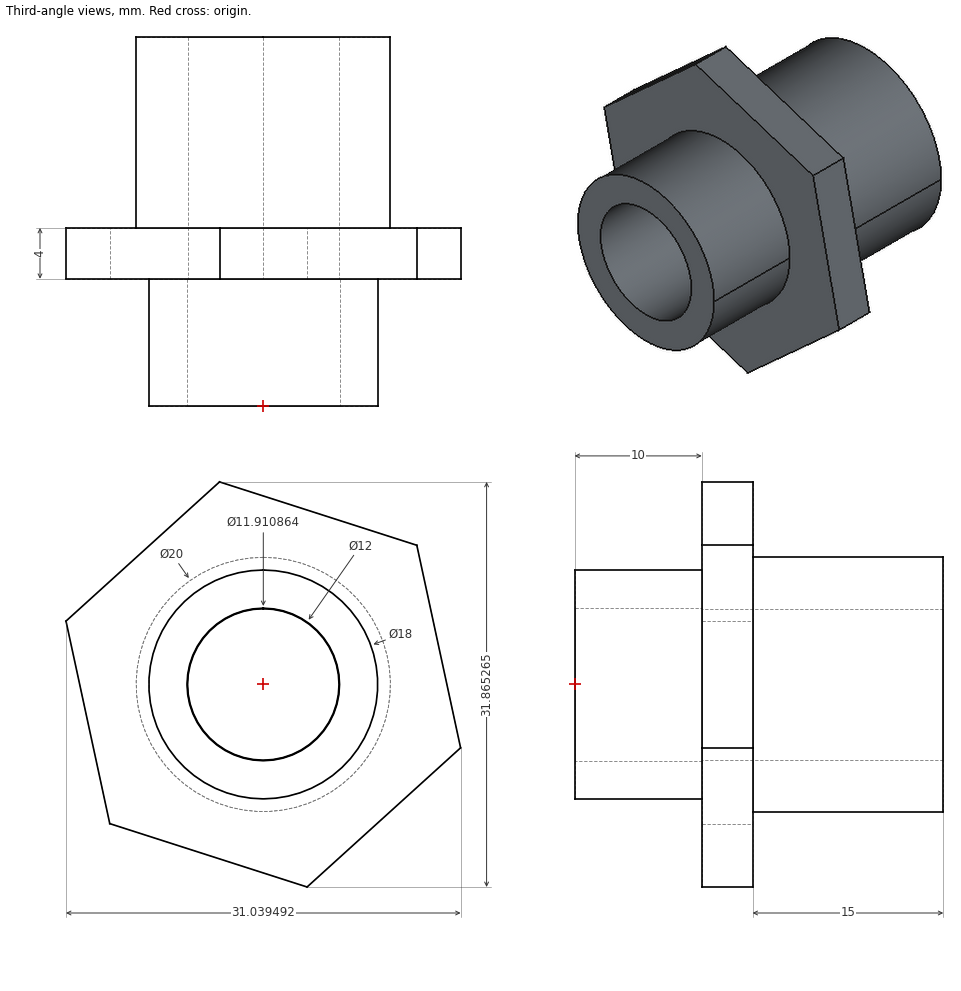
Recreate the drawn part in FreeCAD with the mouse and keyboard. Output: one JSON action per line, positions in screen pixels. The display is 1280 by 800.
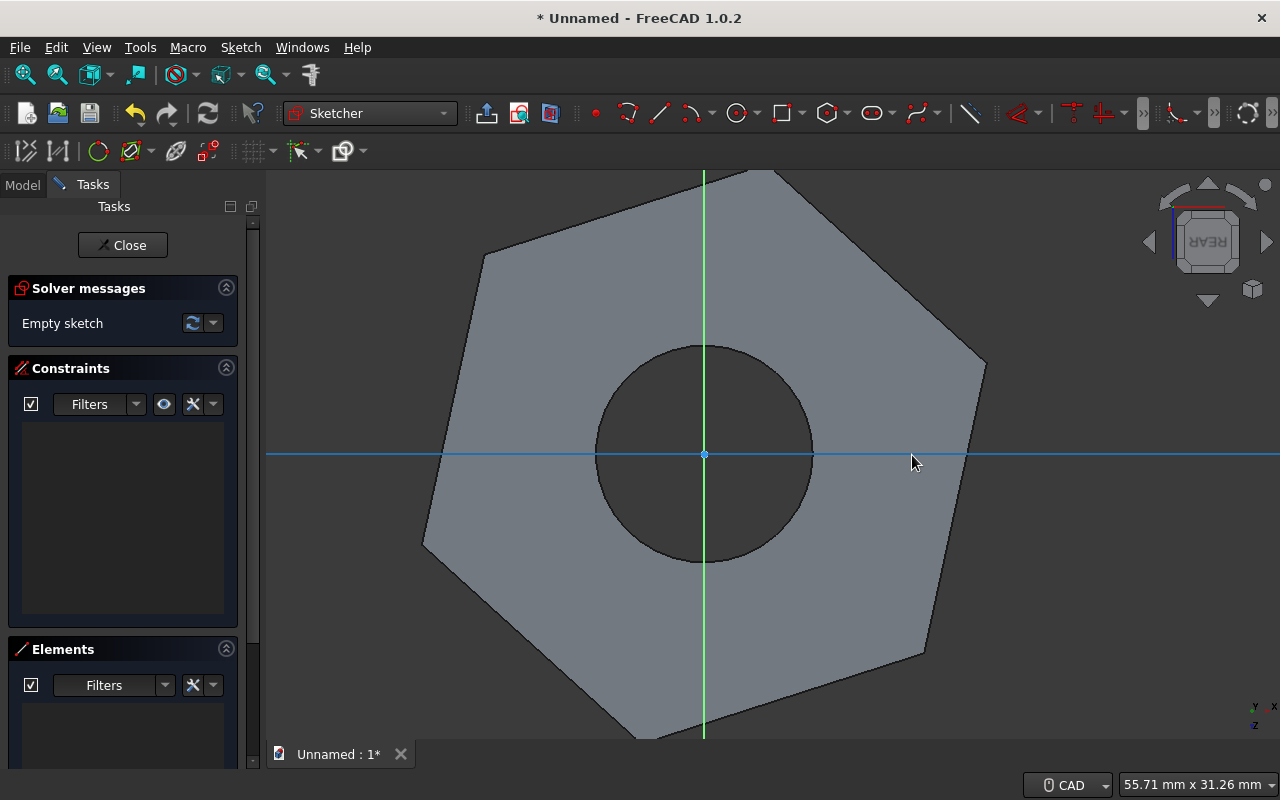
{"action": "left_click", "coordinate": [738, 114]}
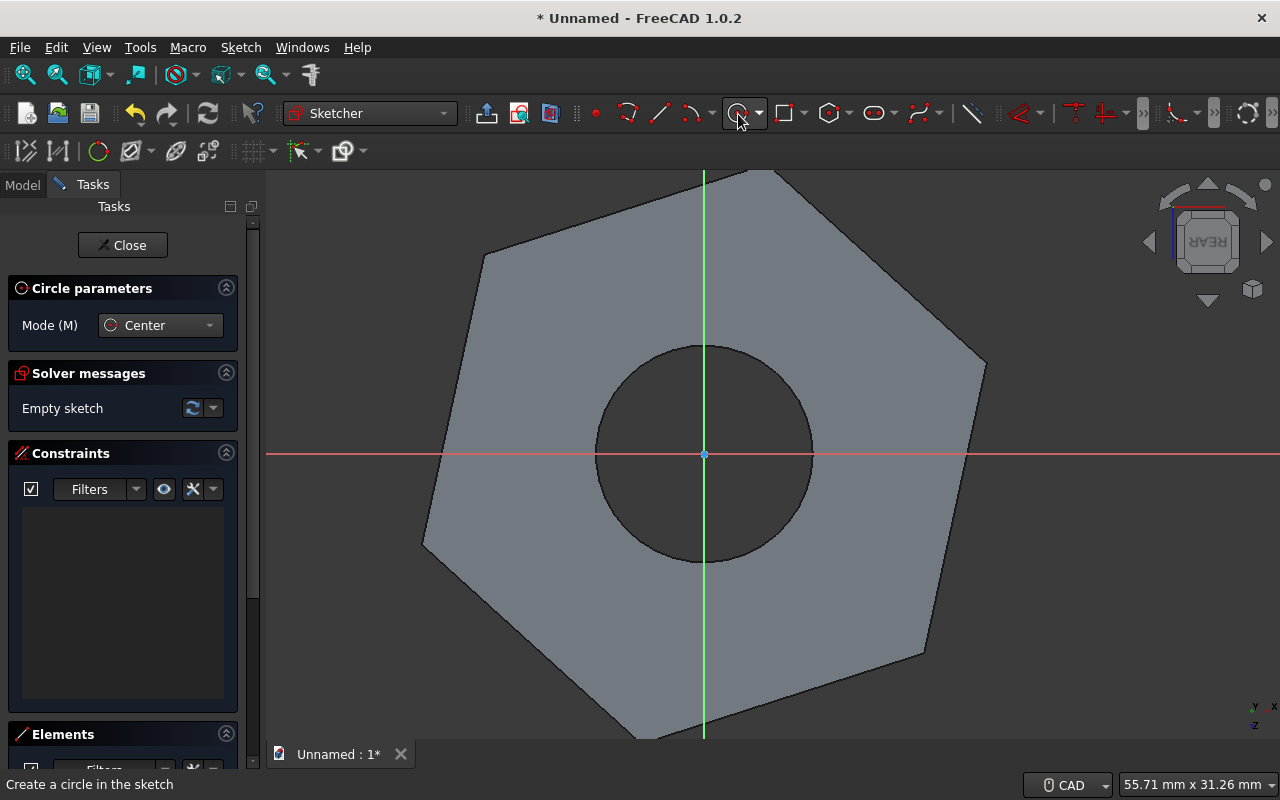
{"action": "left_click", "coordinate": [704, 454]}
{"action": "mouse_move", "coordinate": [833, 325]}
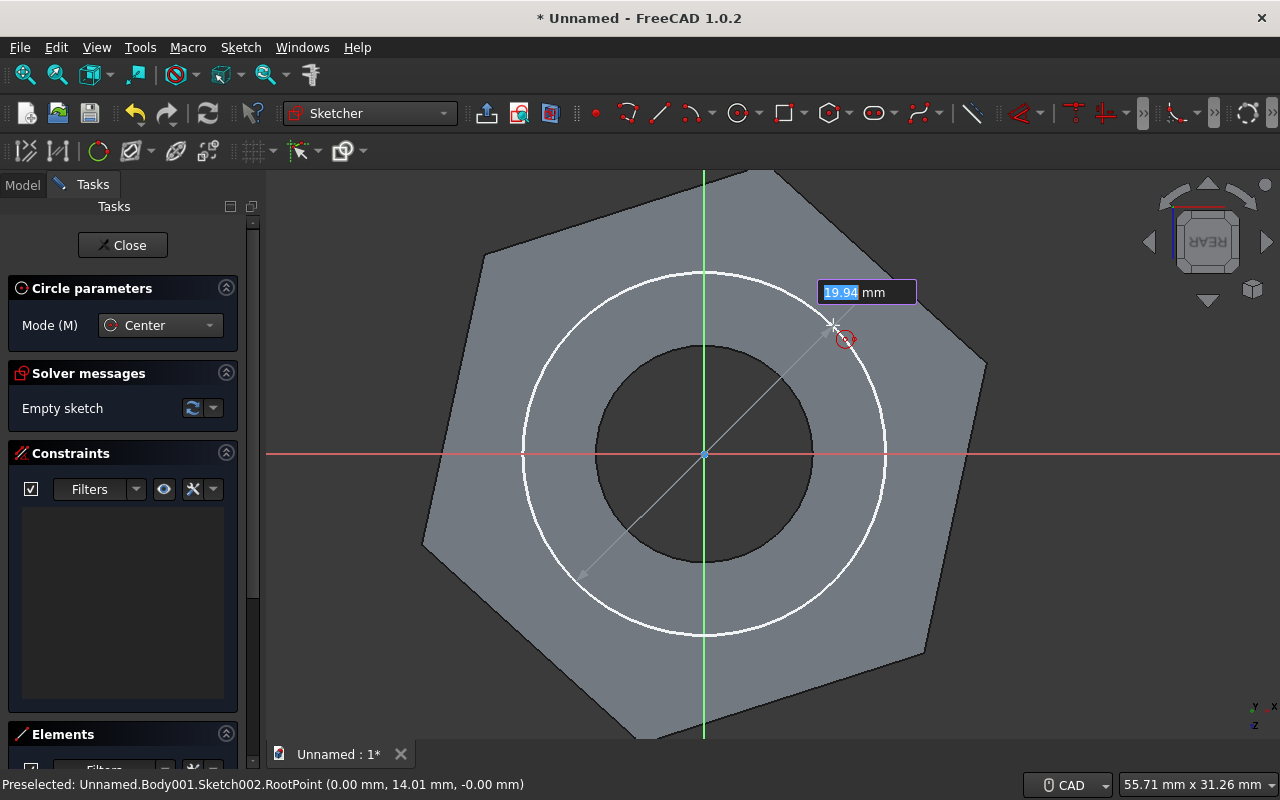
{"action": "type", "text": "20"}
{"action": "key", "text": "Return"}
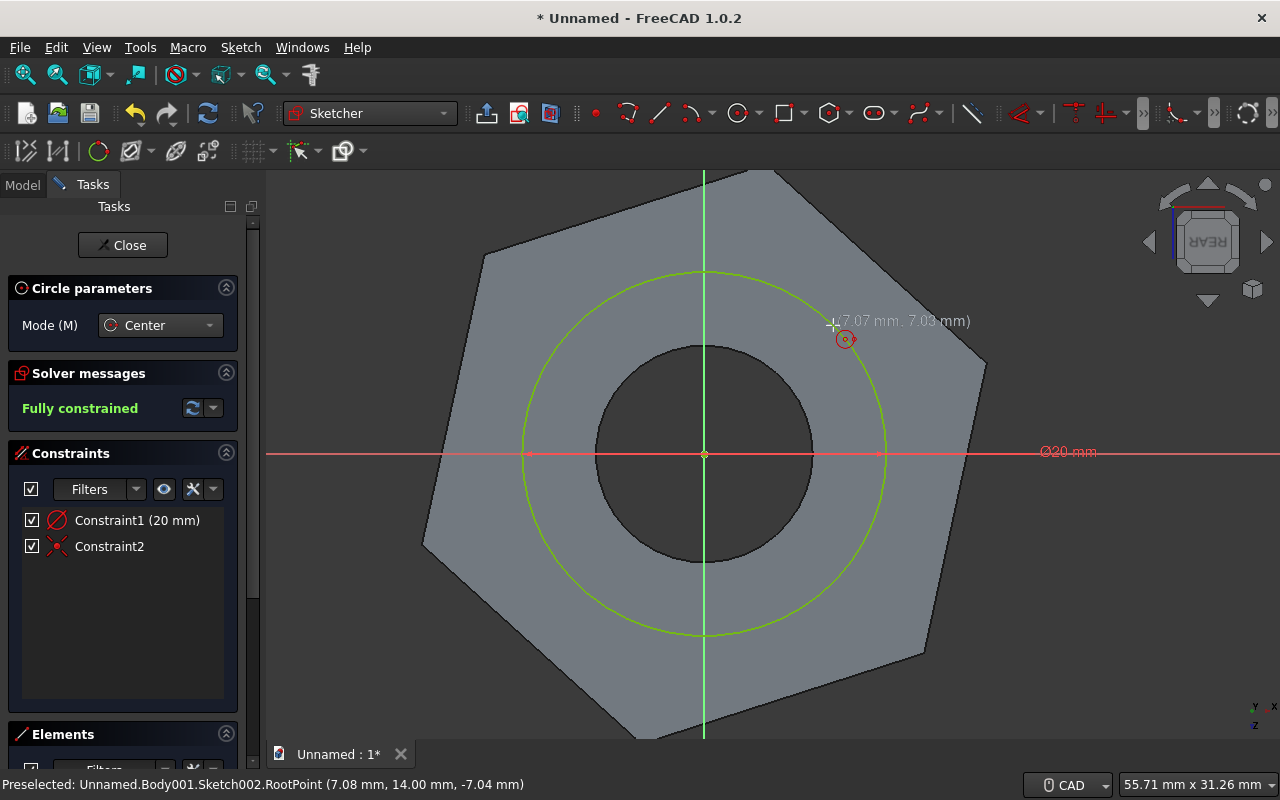
{"action": "left_click", "coordinate": [704, 454]}
{"action": "mouse_move", "coordinate": [781, 377]}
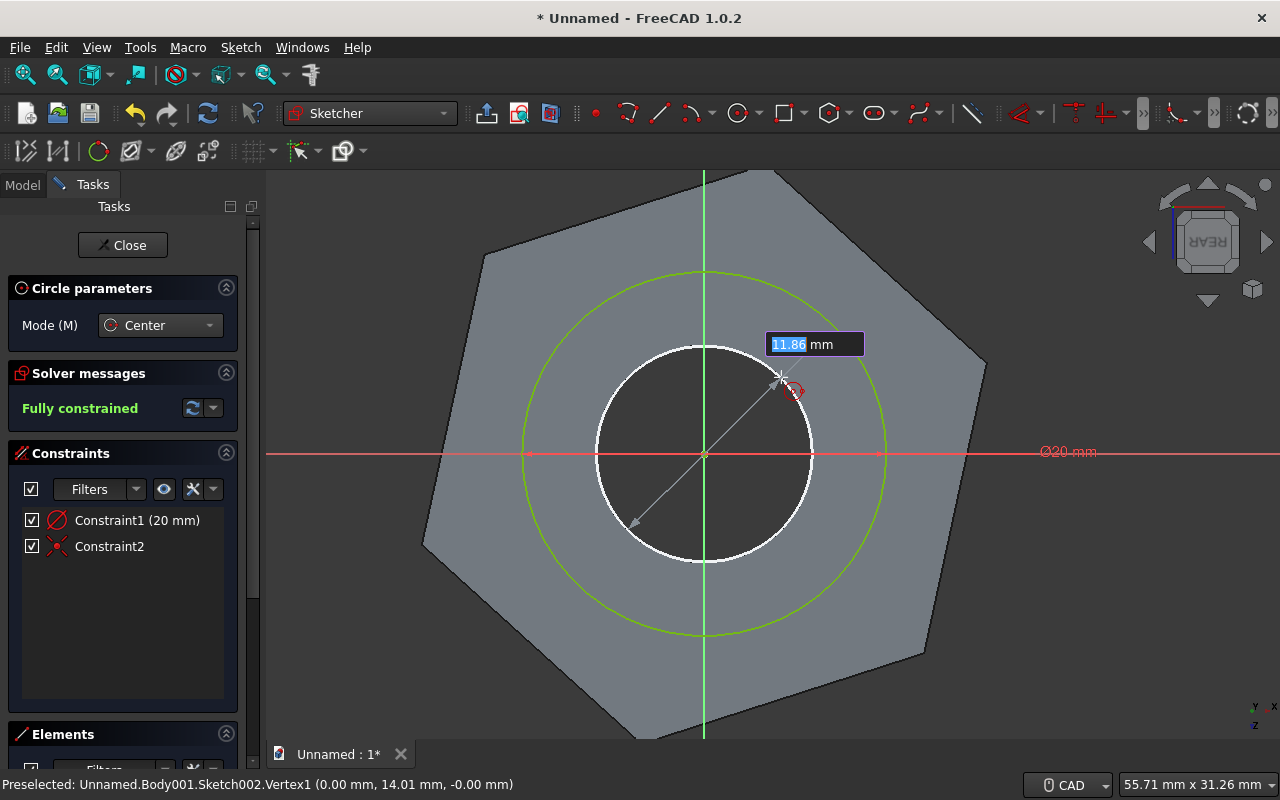
{"action": "type", "text": "11.910864"}
{"action": "key", "text": "Return"}
{"action": "key", "text": "Escape"}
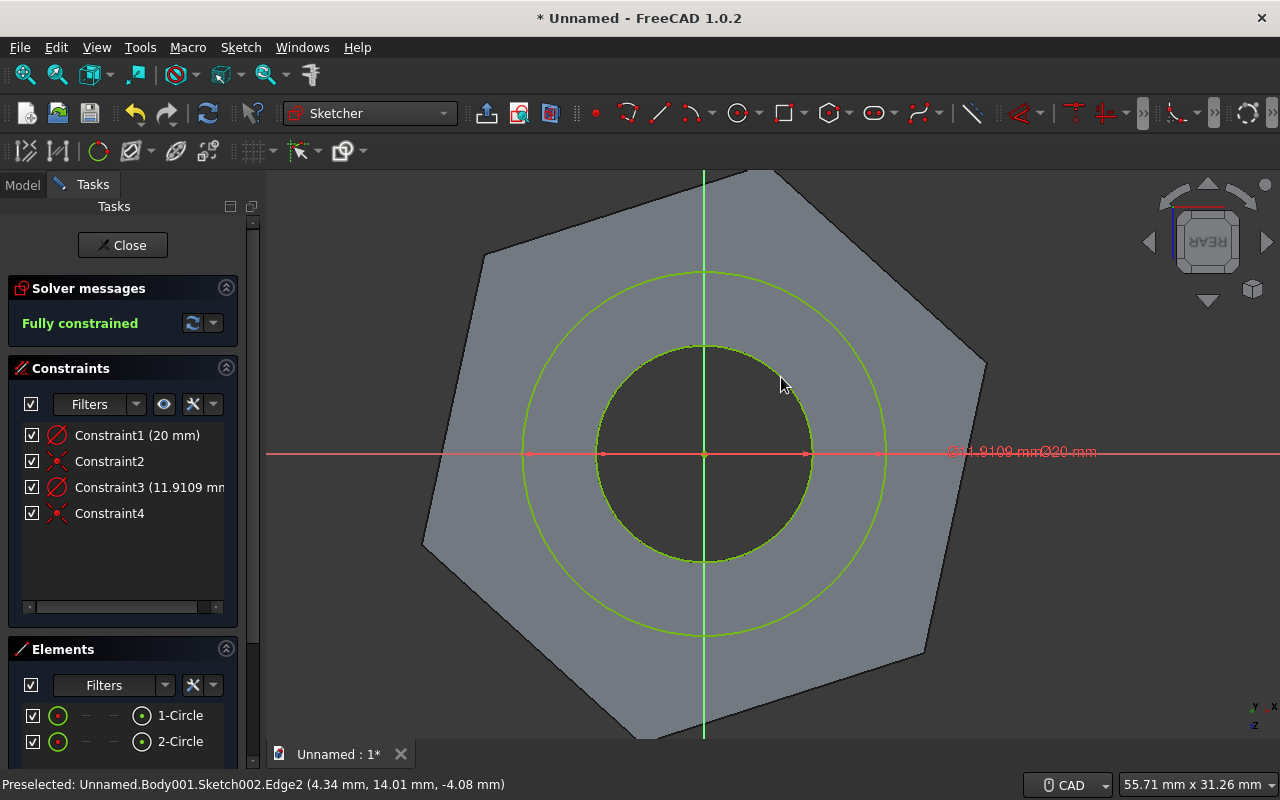
{"action": "left_click", "coordinate": [123, 245]}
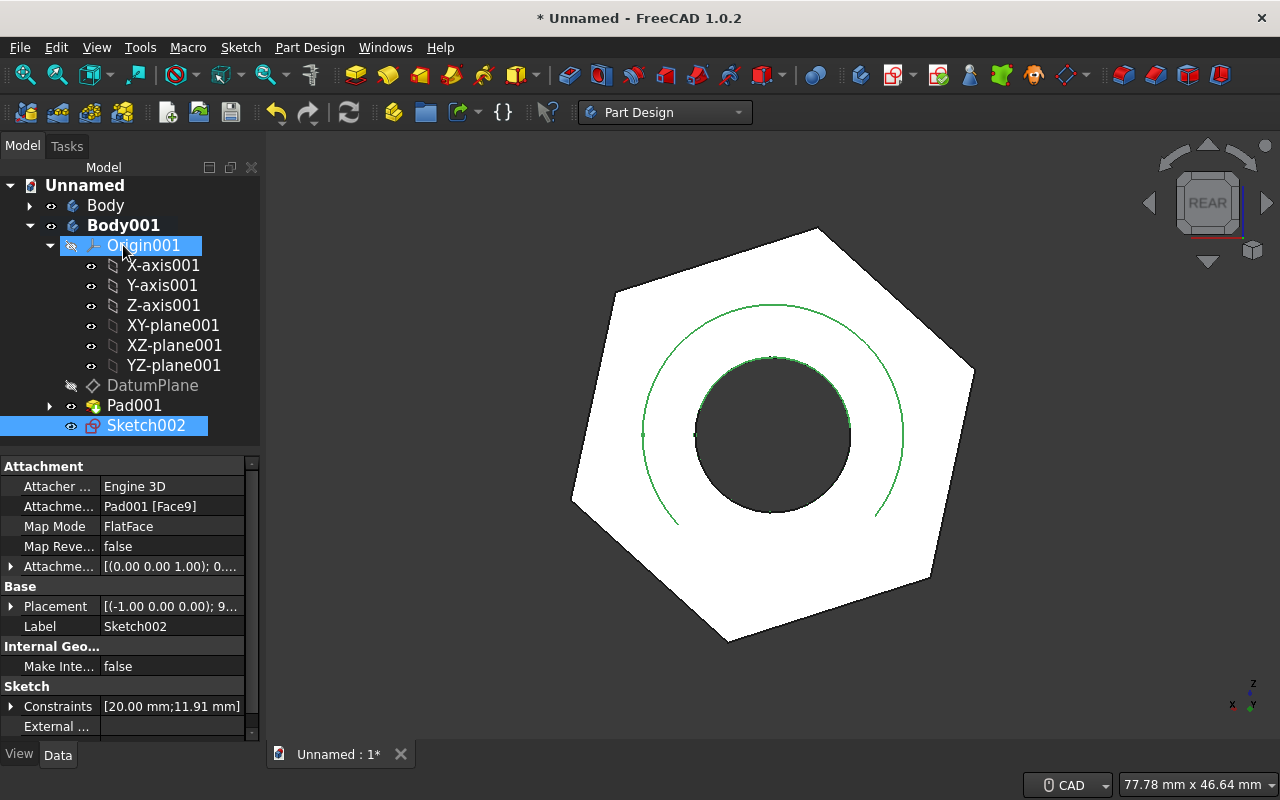
{"action": "left_click", "coordinate": [356, 76]}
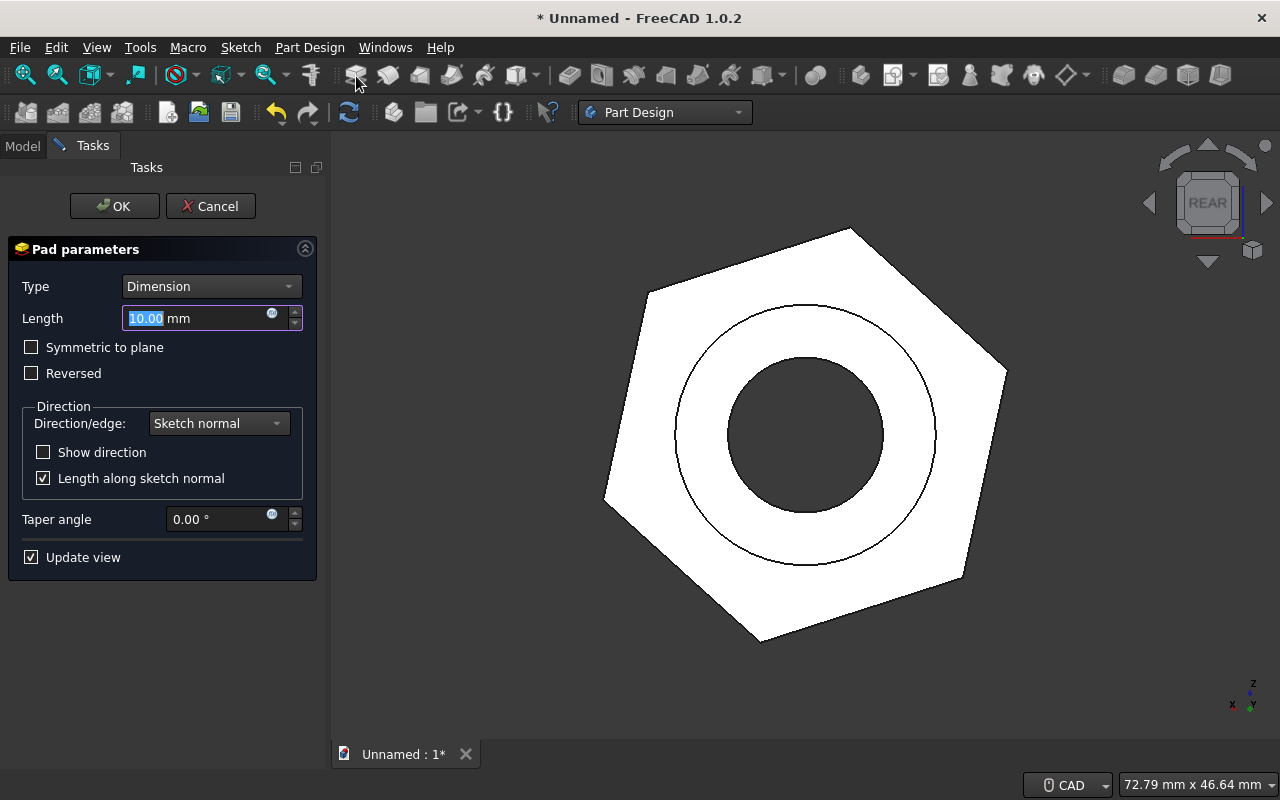
{"action": "type", "text": "15"}
{"action": "key", "text": "Tab"}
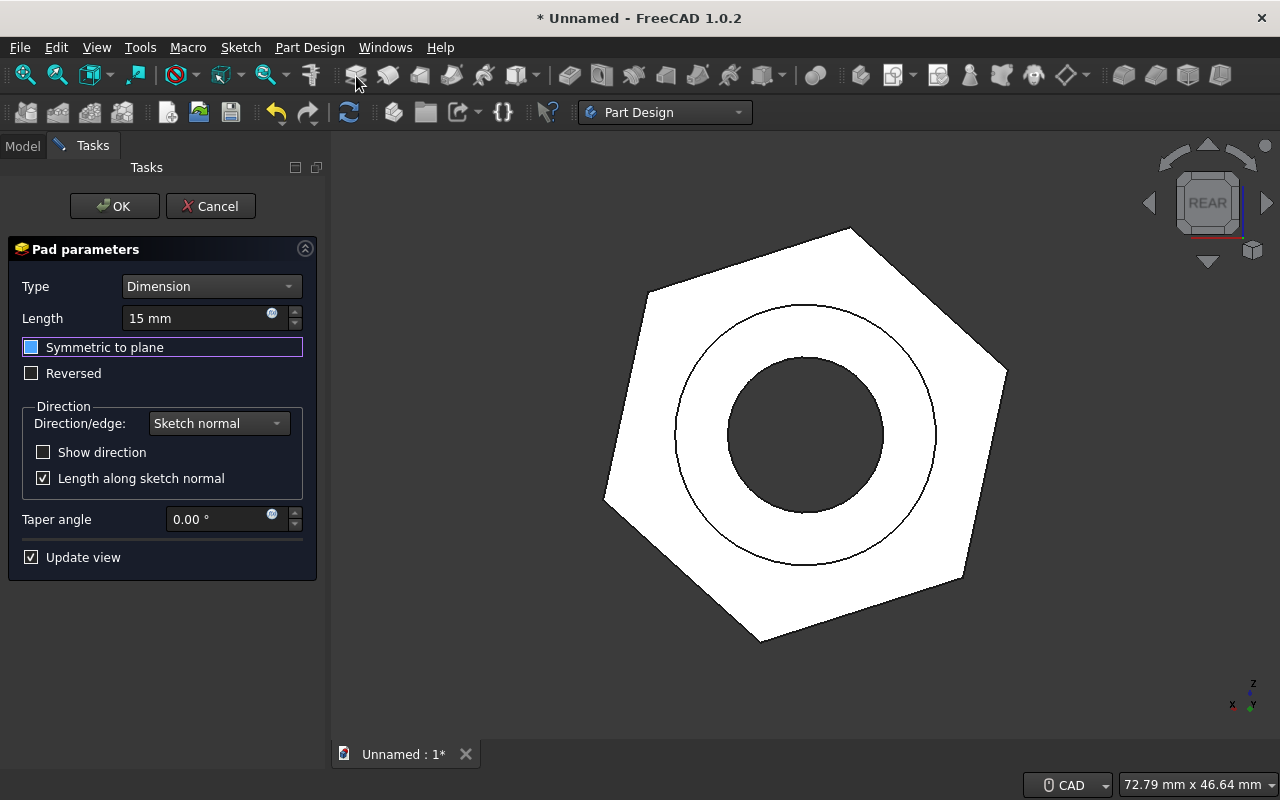
{"action": "left_click", "coordinate": [115, 206]}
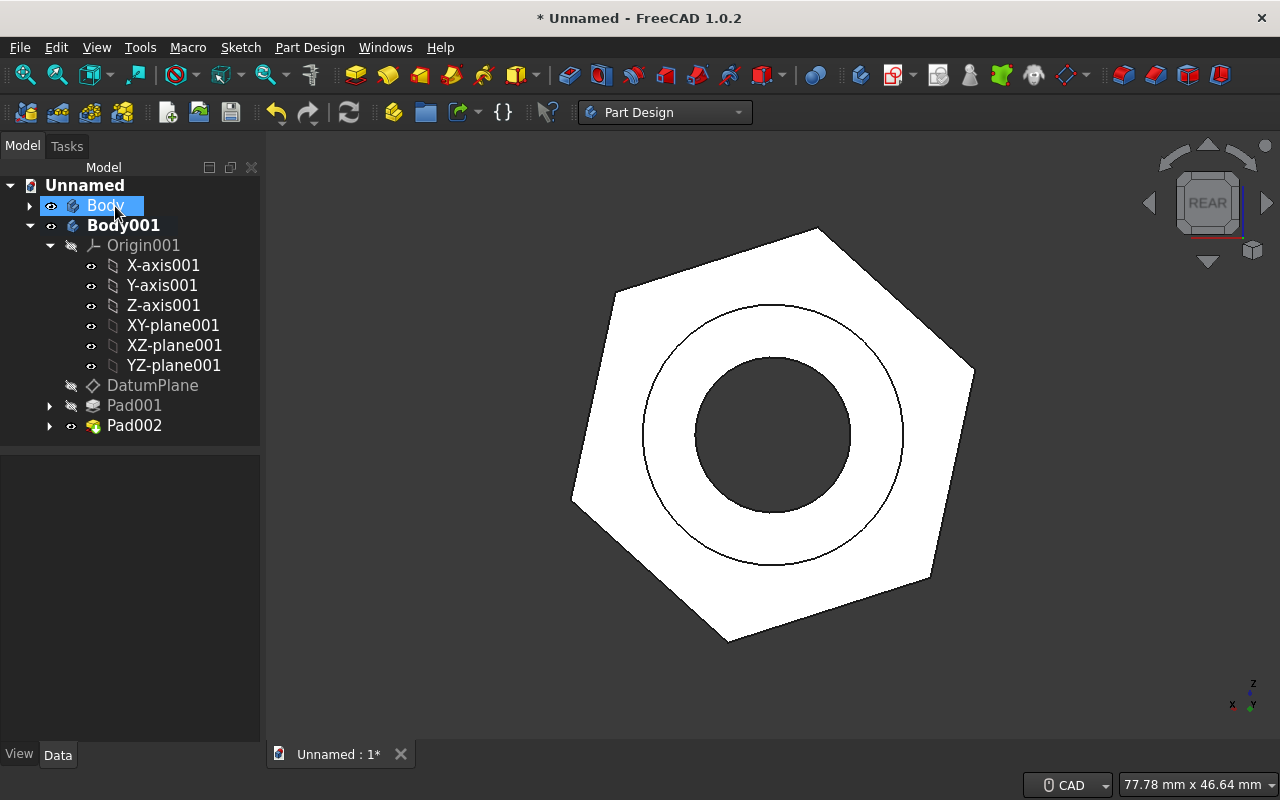
{"action": "key", "text": "0"}